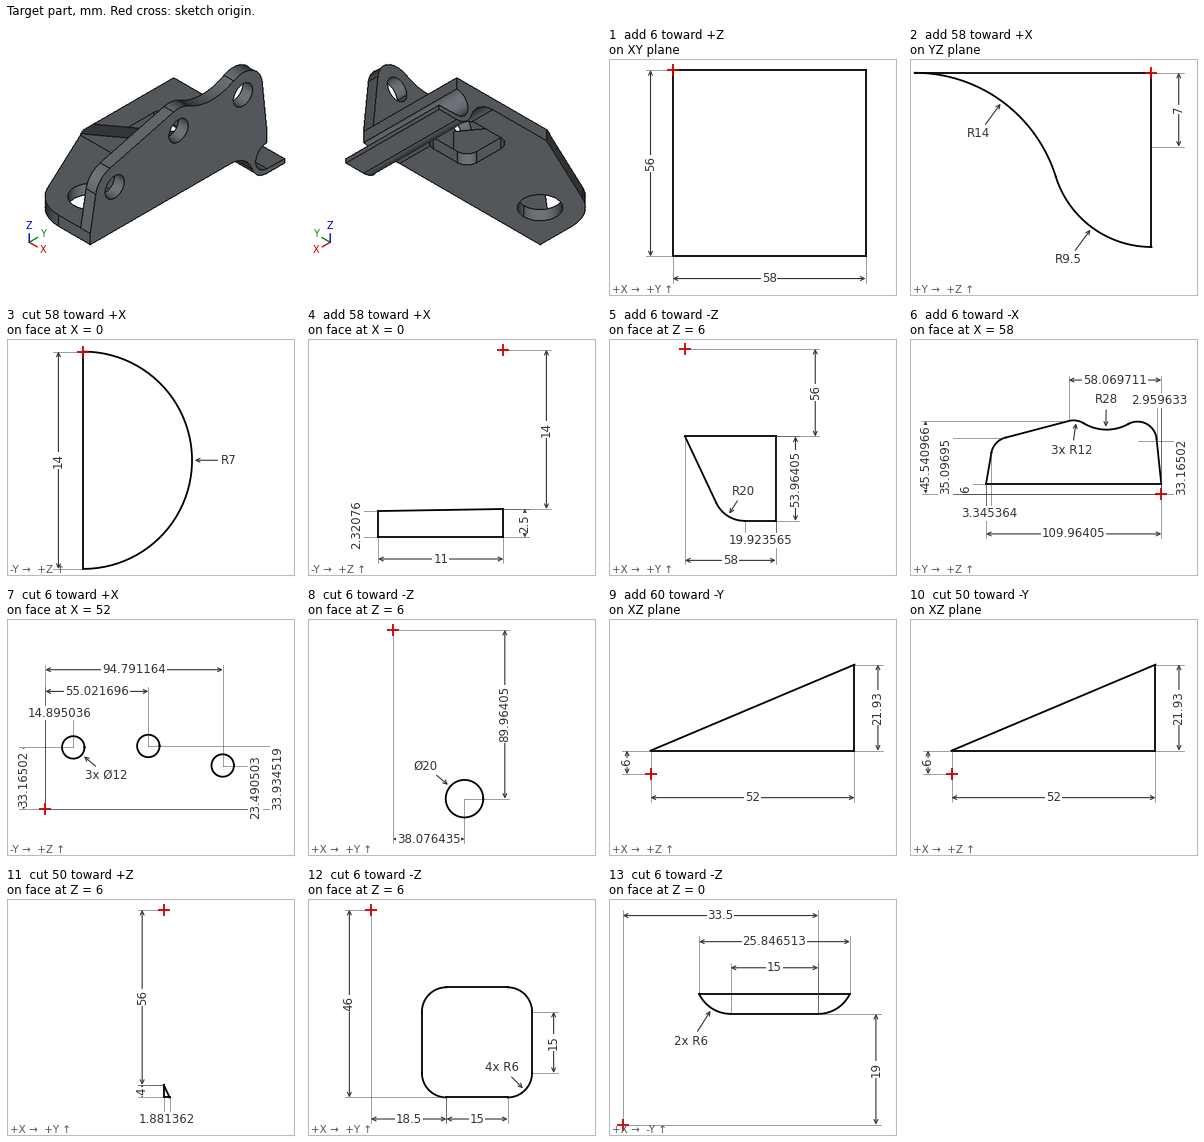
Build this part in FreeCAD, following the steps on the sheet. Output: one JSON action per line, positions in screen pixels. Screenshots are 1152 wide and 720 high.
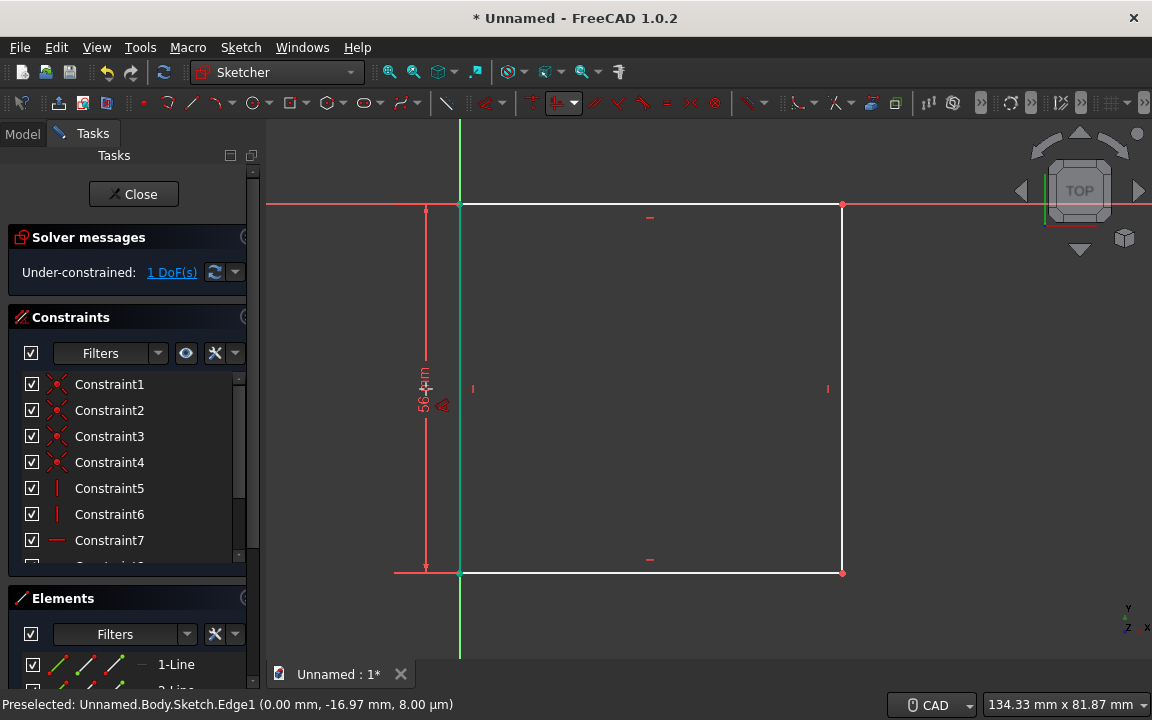
{"action": "left_click", "coordinate": [574, 573]}
{"action": "left_click", "coordinate": [651, 607]}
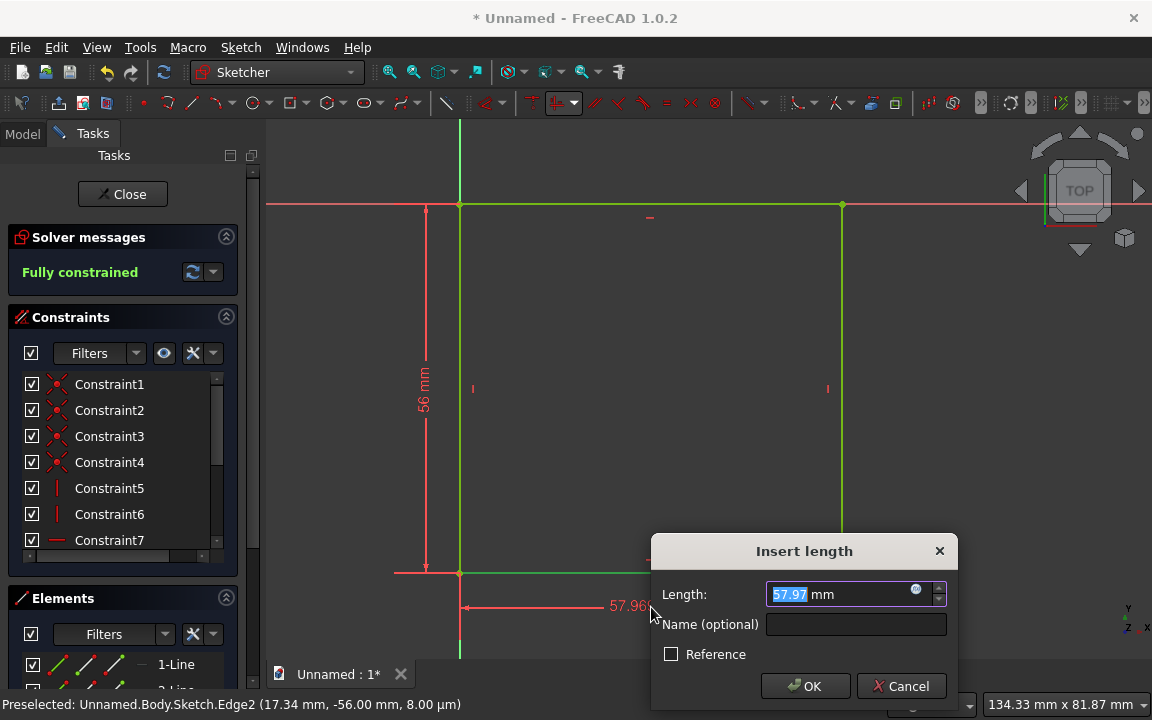
{"action": "type", "text": "58"}
{"action": "key", "text": "Return"}
{"action": "key", "text": "Escape"}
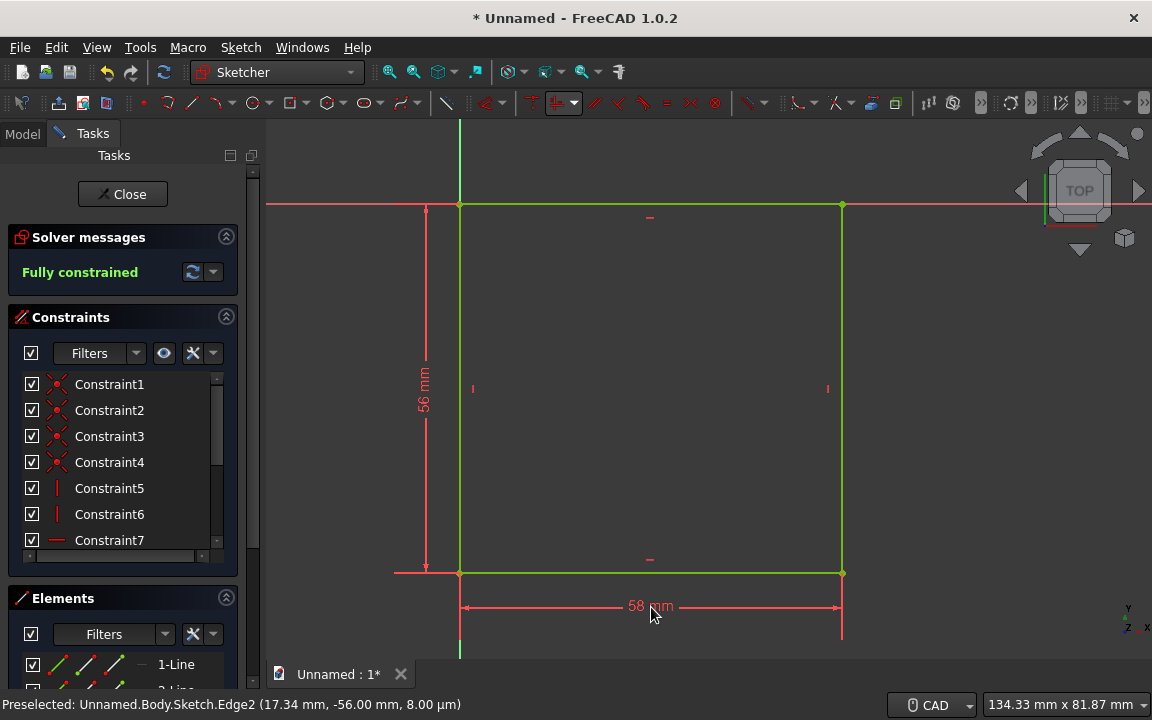
{"action": "left_click", "coordinate": [123, 194]}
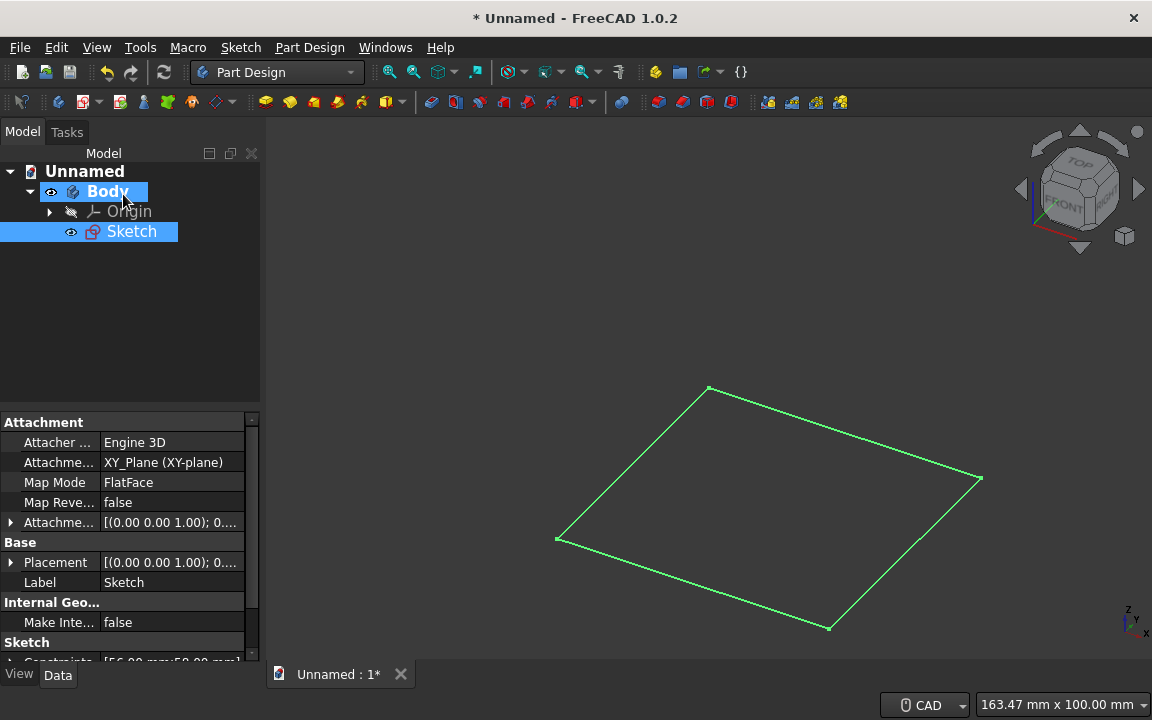
{"action": "left_click", "coordinate": [266, 102]}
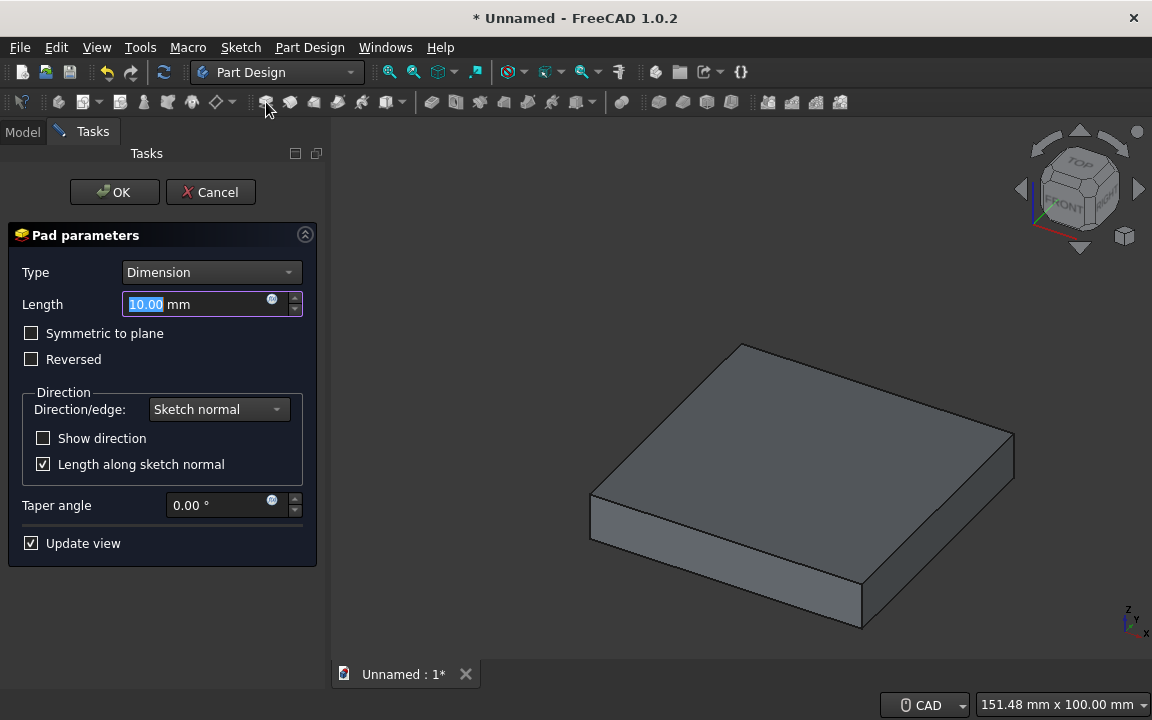
{"action": "type", "text": "6"}
{"action": "key", "text": "Tab"}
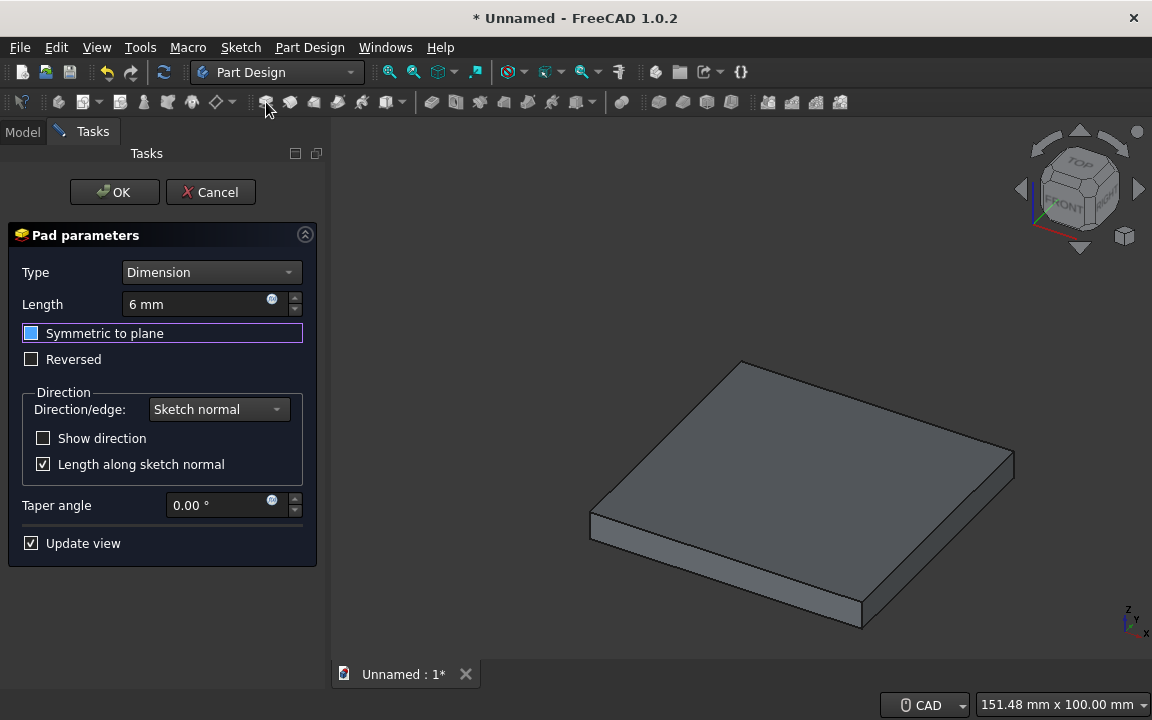
{"action": "left_click", "coordinate": [115, 192]}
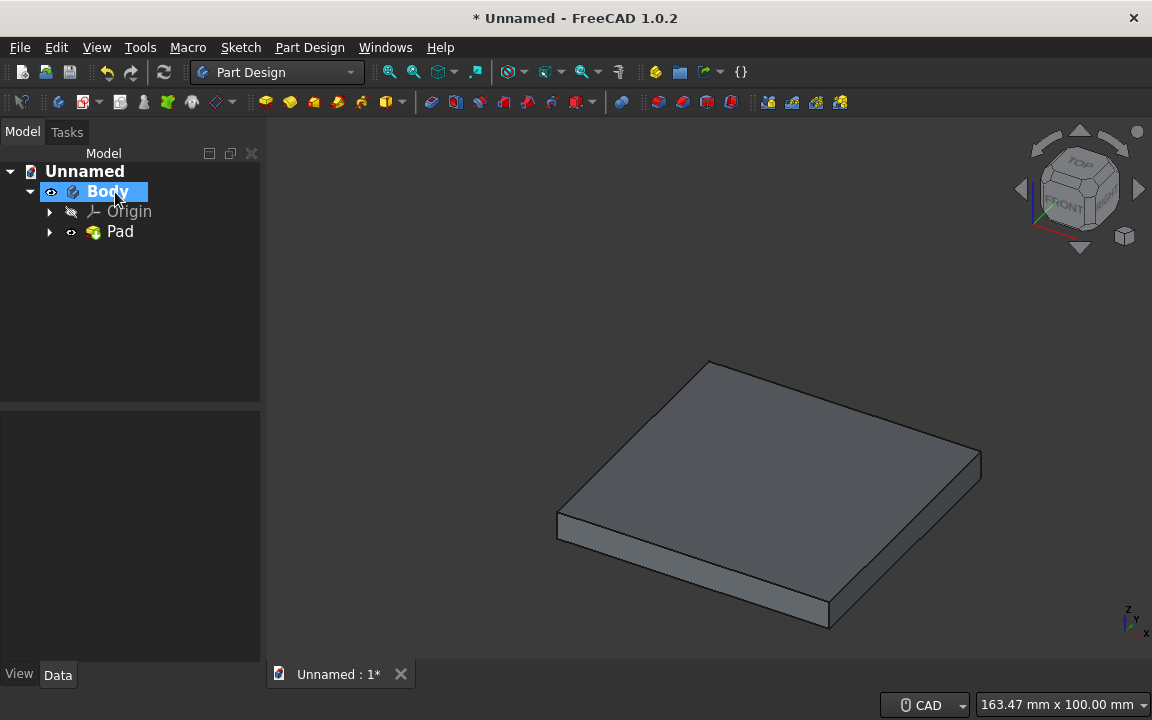
{"action": "left_click", "coordinate": [84, 102]}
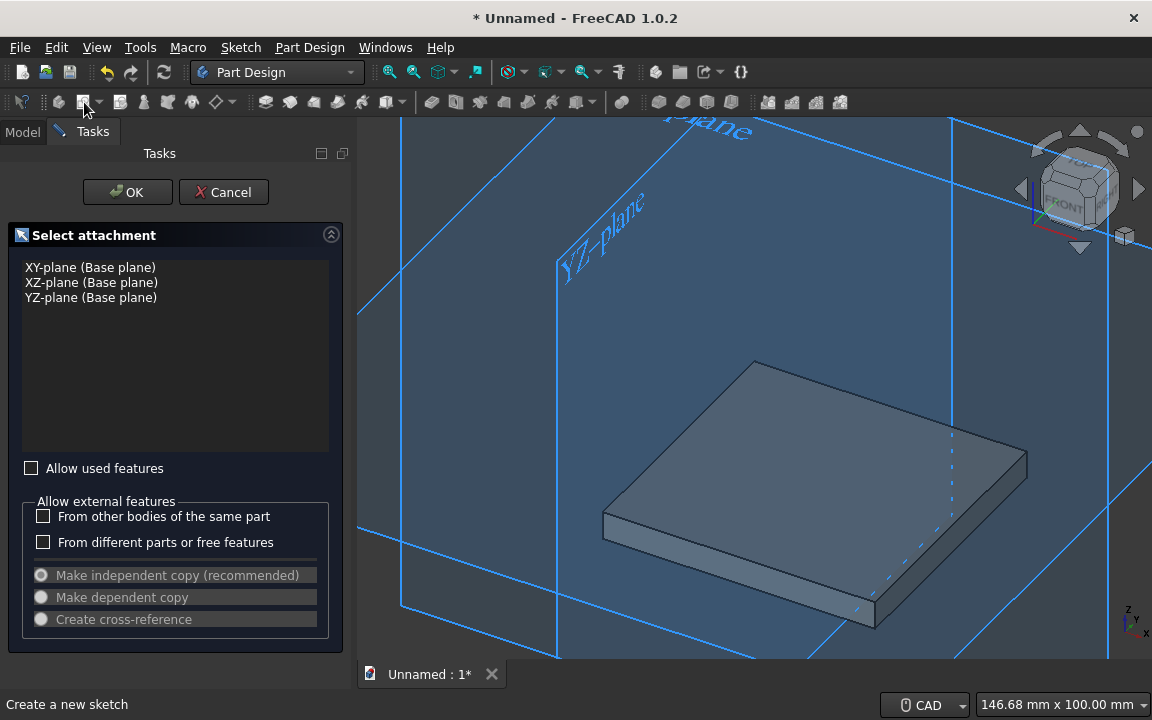
{"action": "left_click", "coordinate": [82, 298]}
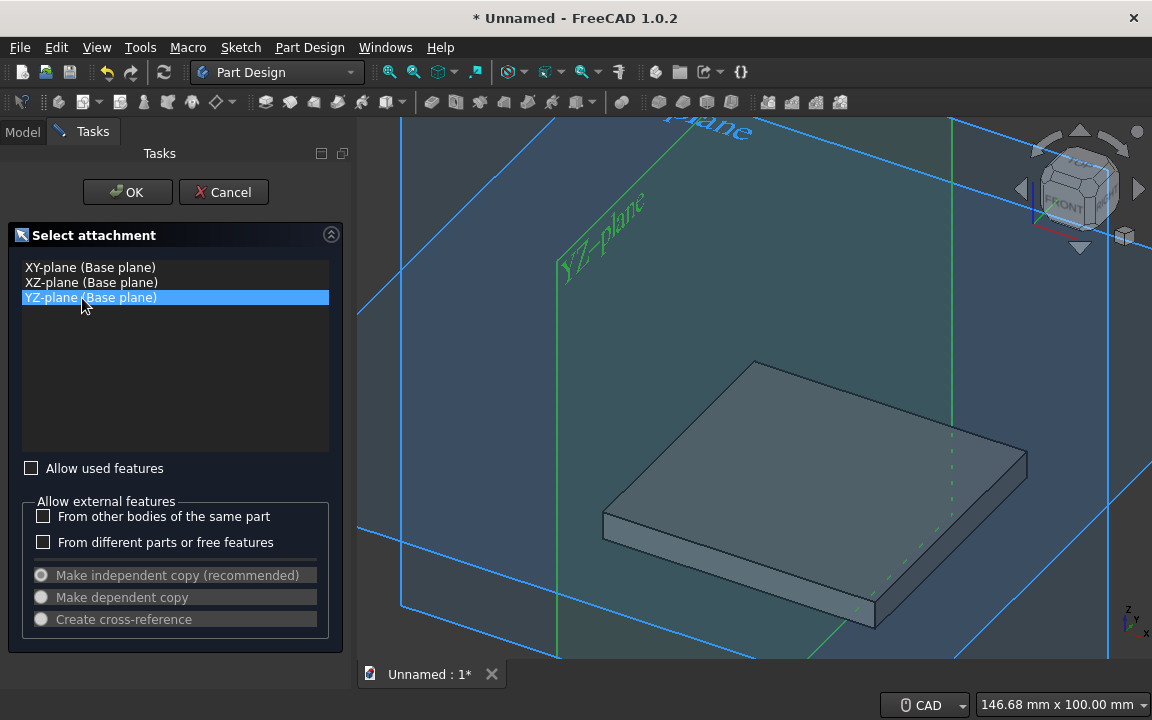
{"action": "left_click", "coordinate": [128, 192]}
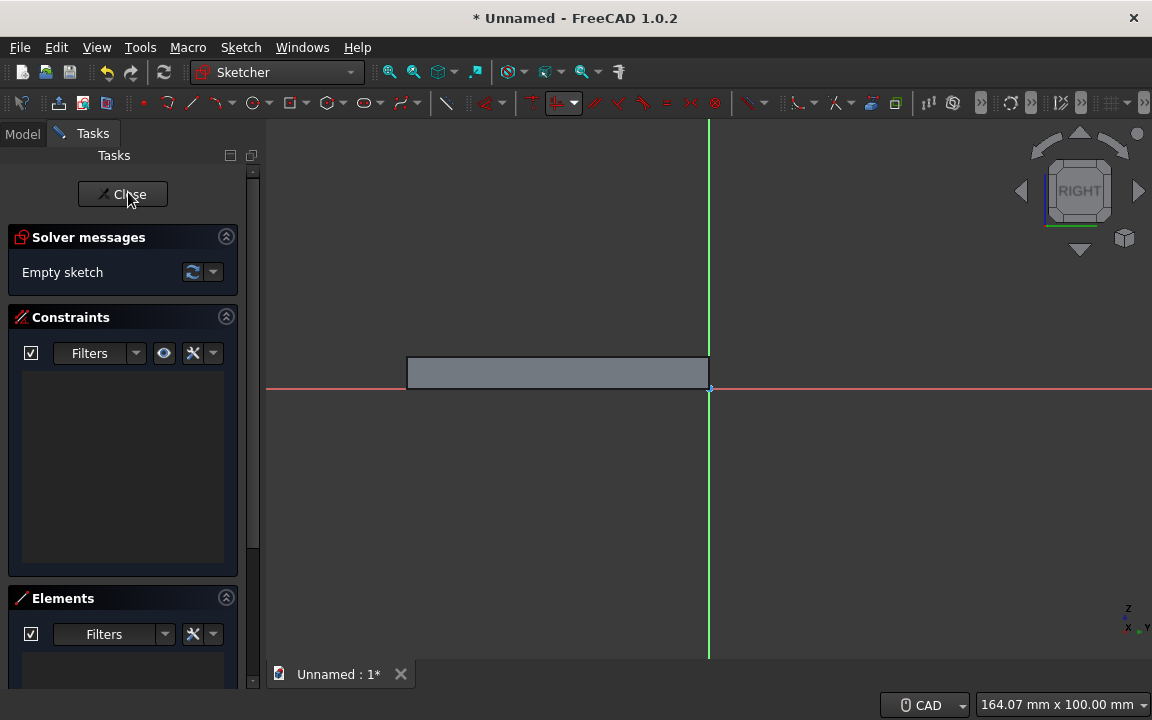
{"action": "left_click", "coordinate": [108, 104]}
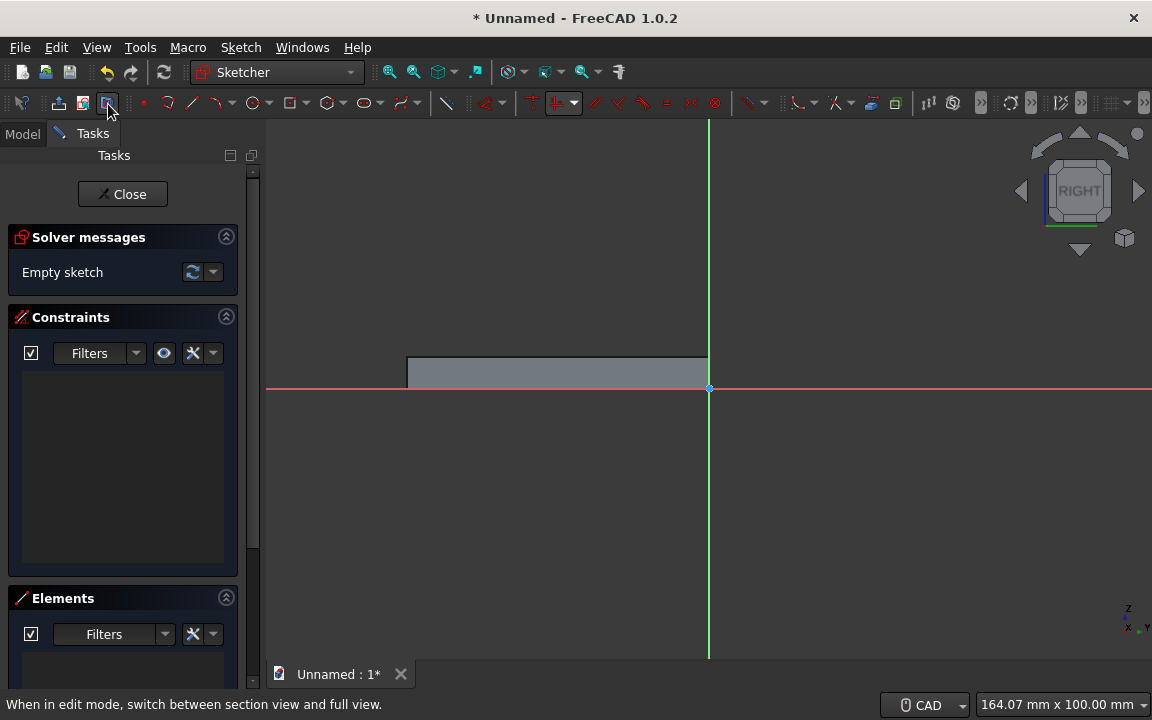
{"action": "scroll", "coordinate": [651, 448], "scroll_direction": "up", "scroll_amount": 7}